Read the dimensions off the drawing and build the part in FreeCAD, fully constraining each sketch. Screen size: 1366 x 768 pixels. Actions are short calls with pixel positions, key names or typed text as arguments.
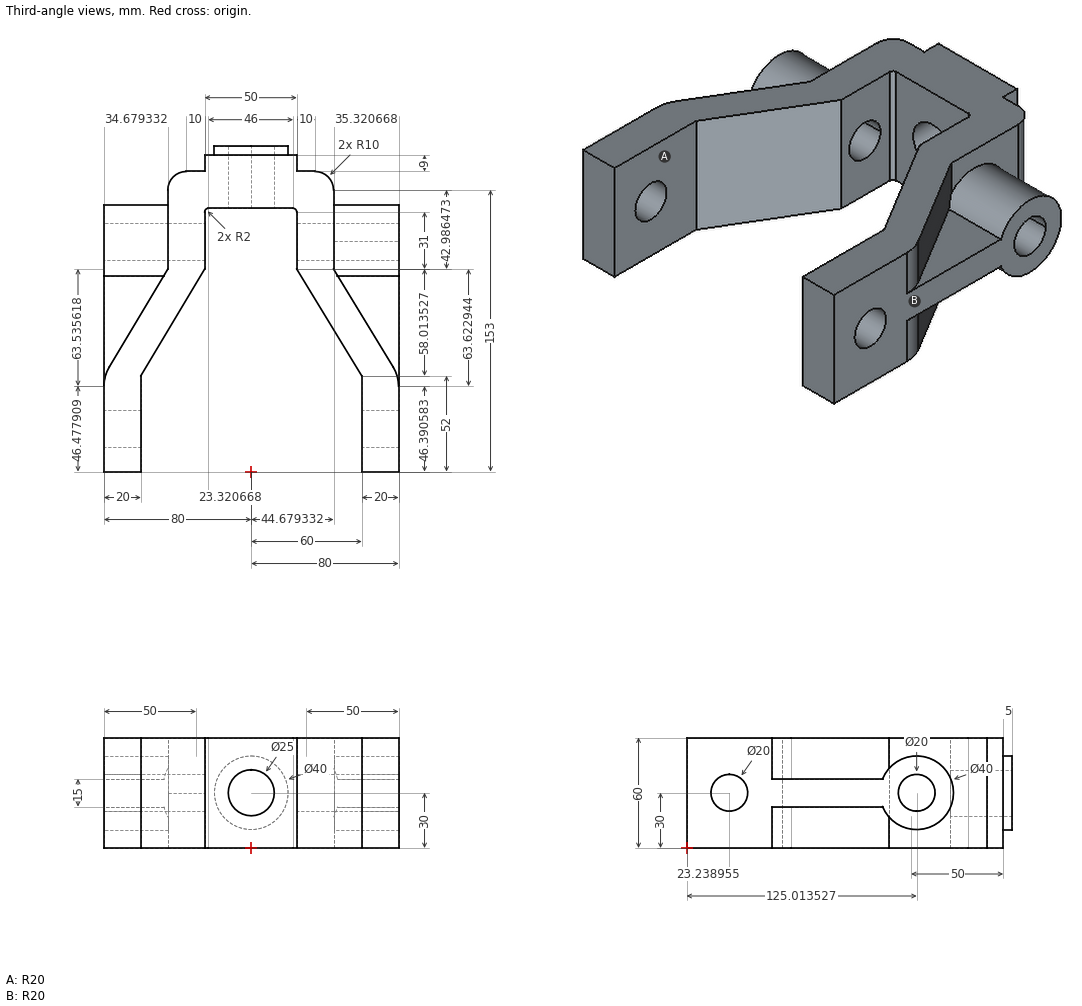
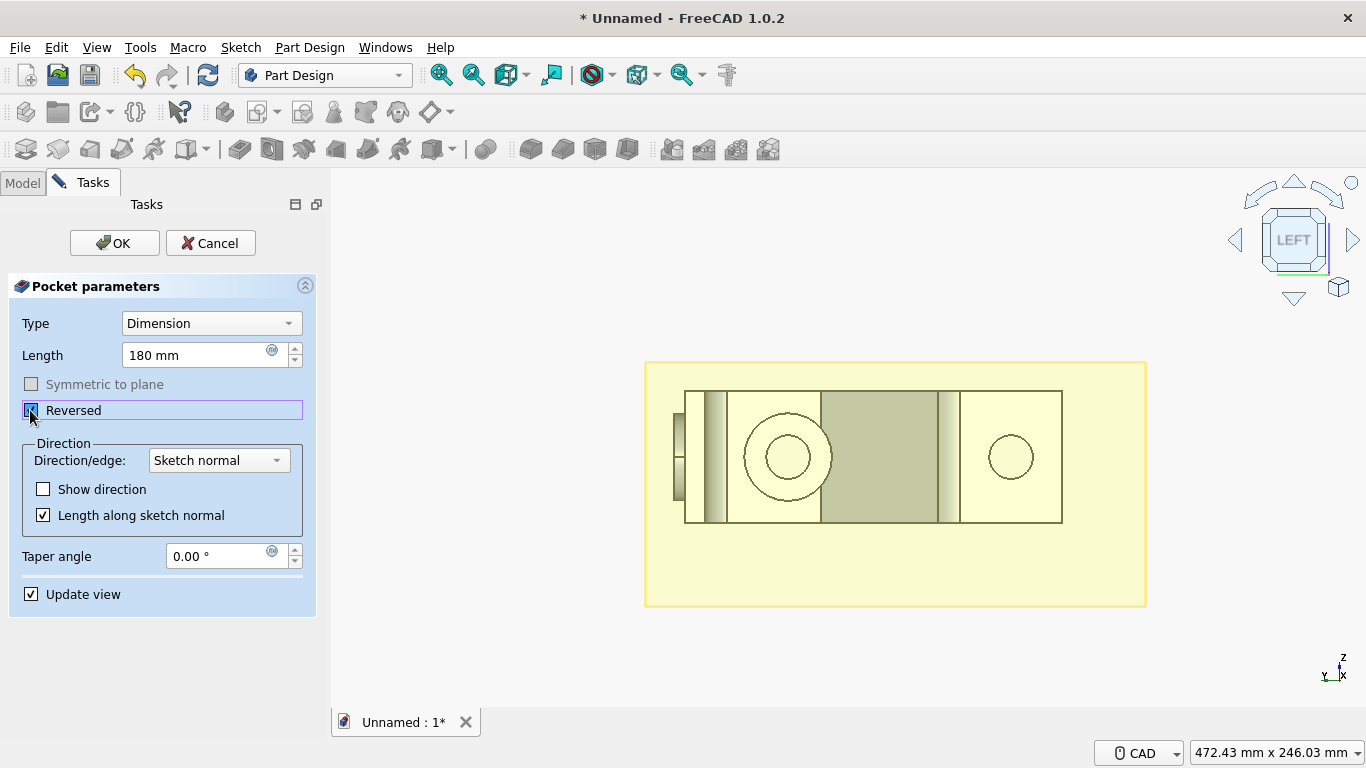
click(115, 243)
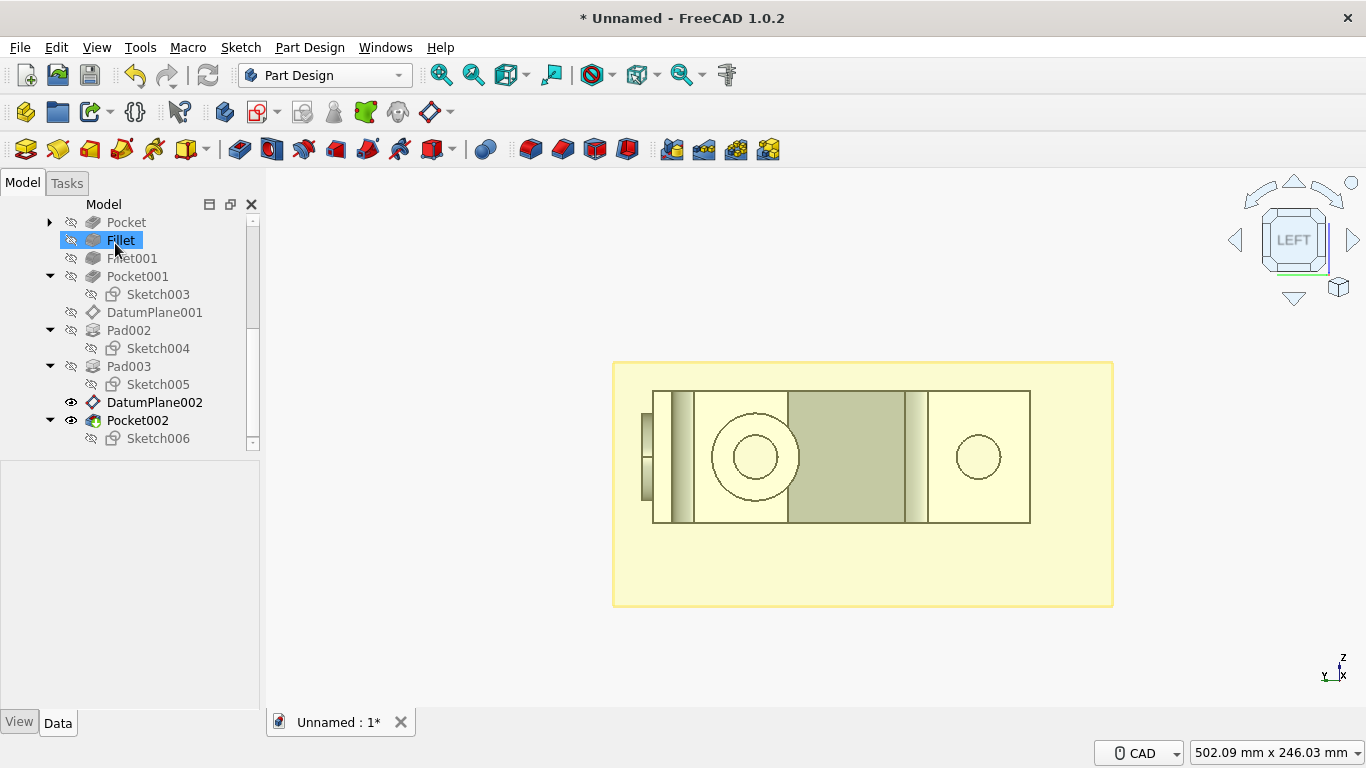
click(116, 402)
key(space)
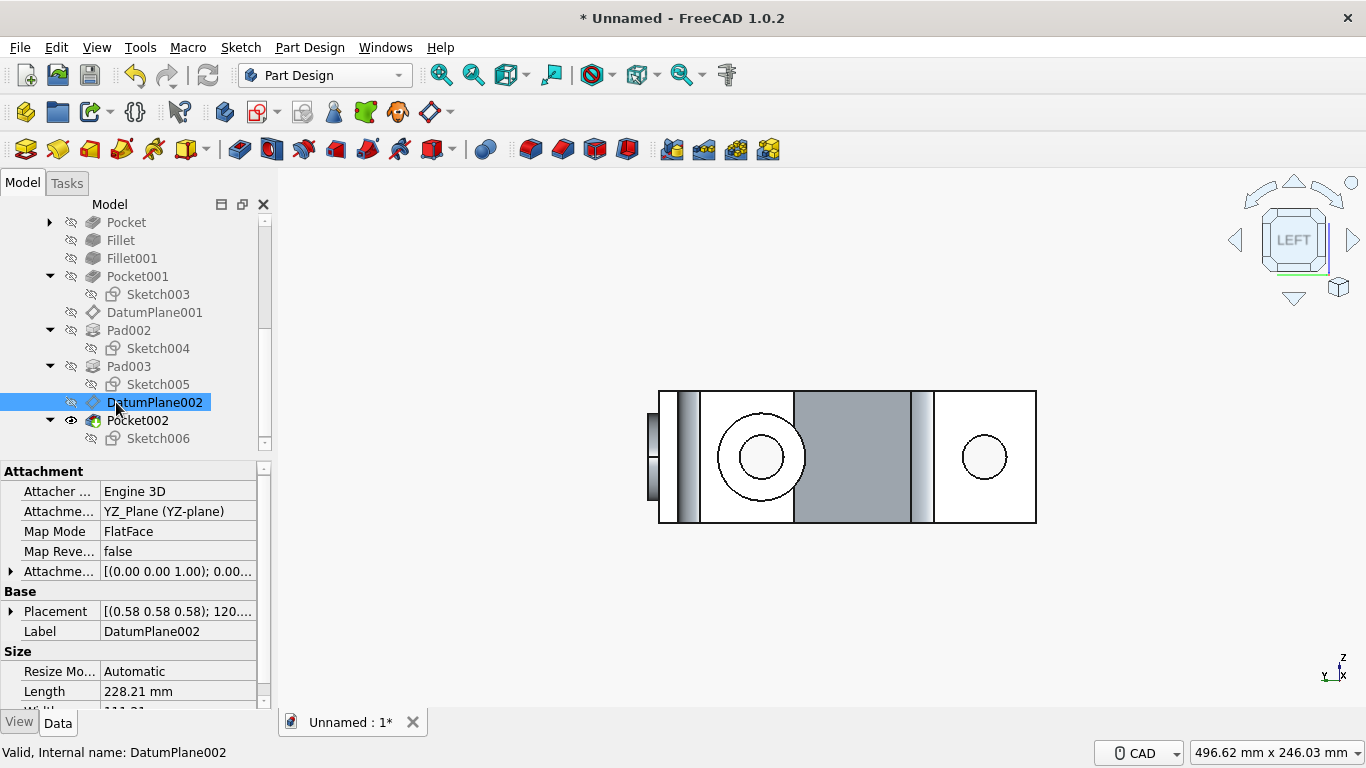
key(v)
key(f)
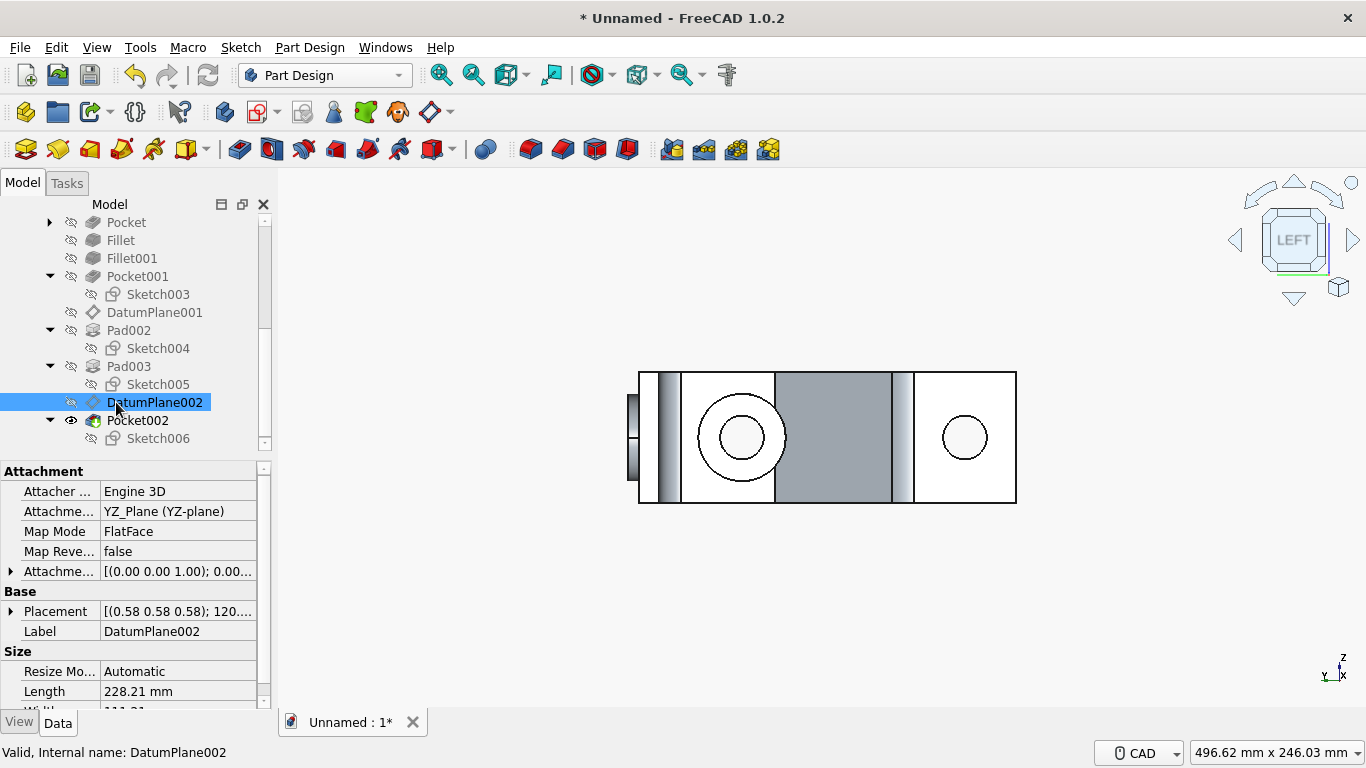
scroll(140, 326, down, 3)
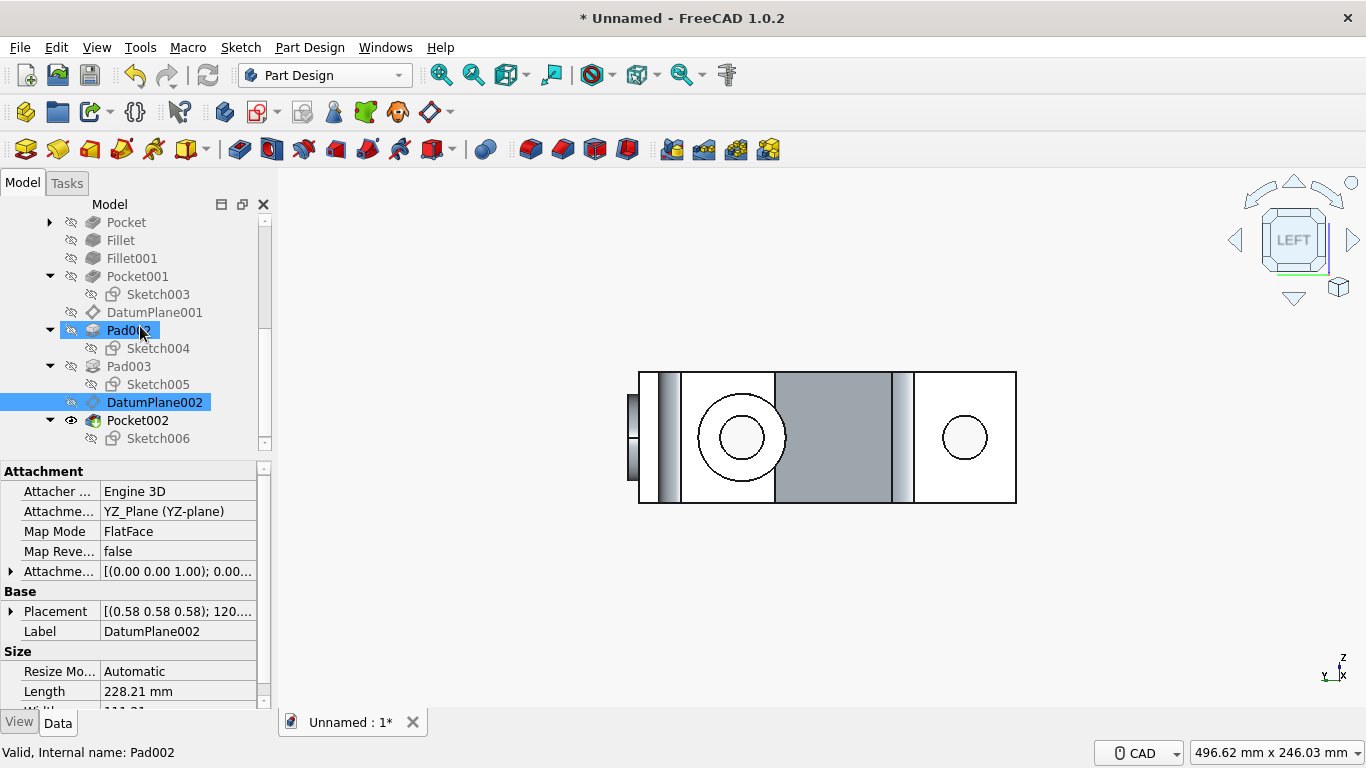
scroll(140, 326, up, 15)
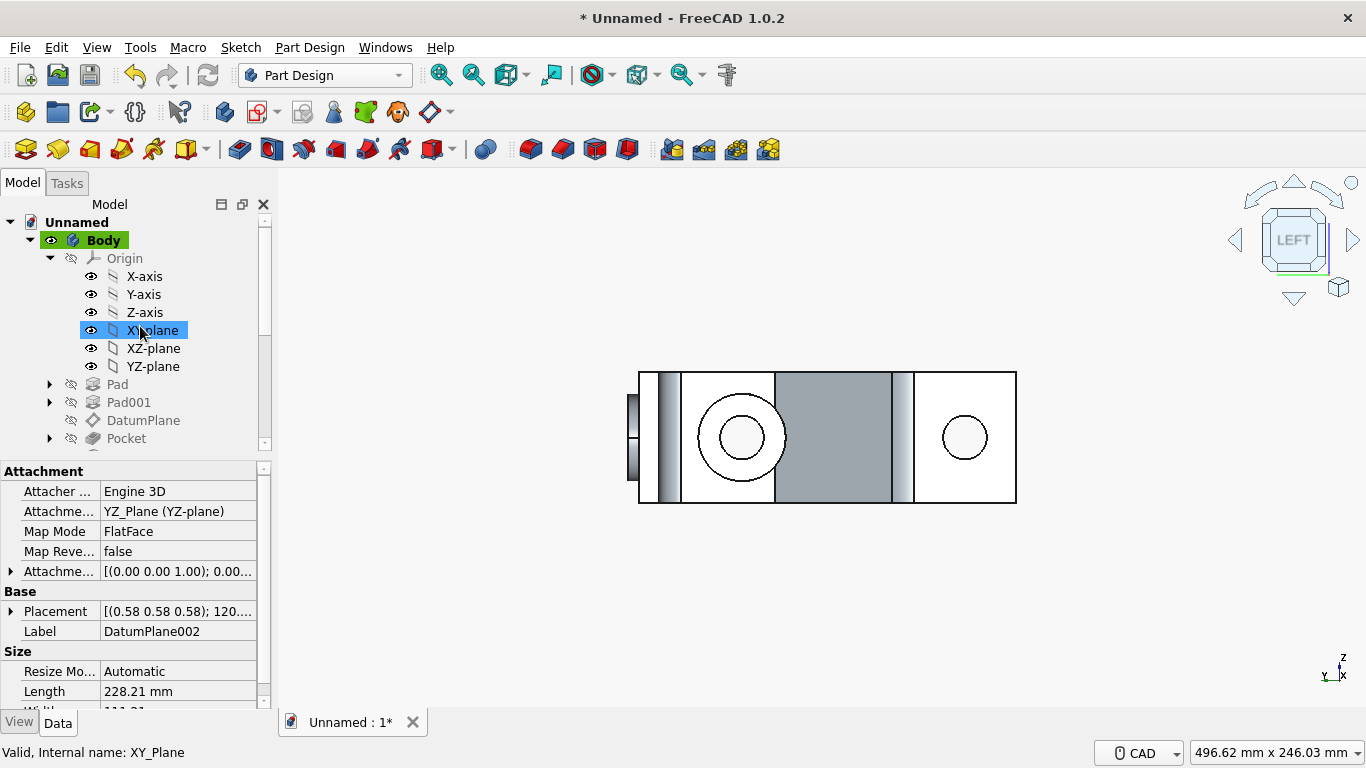
click(136, 330)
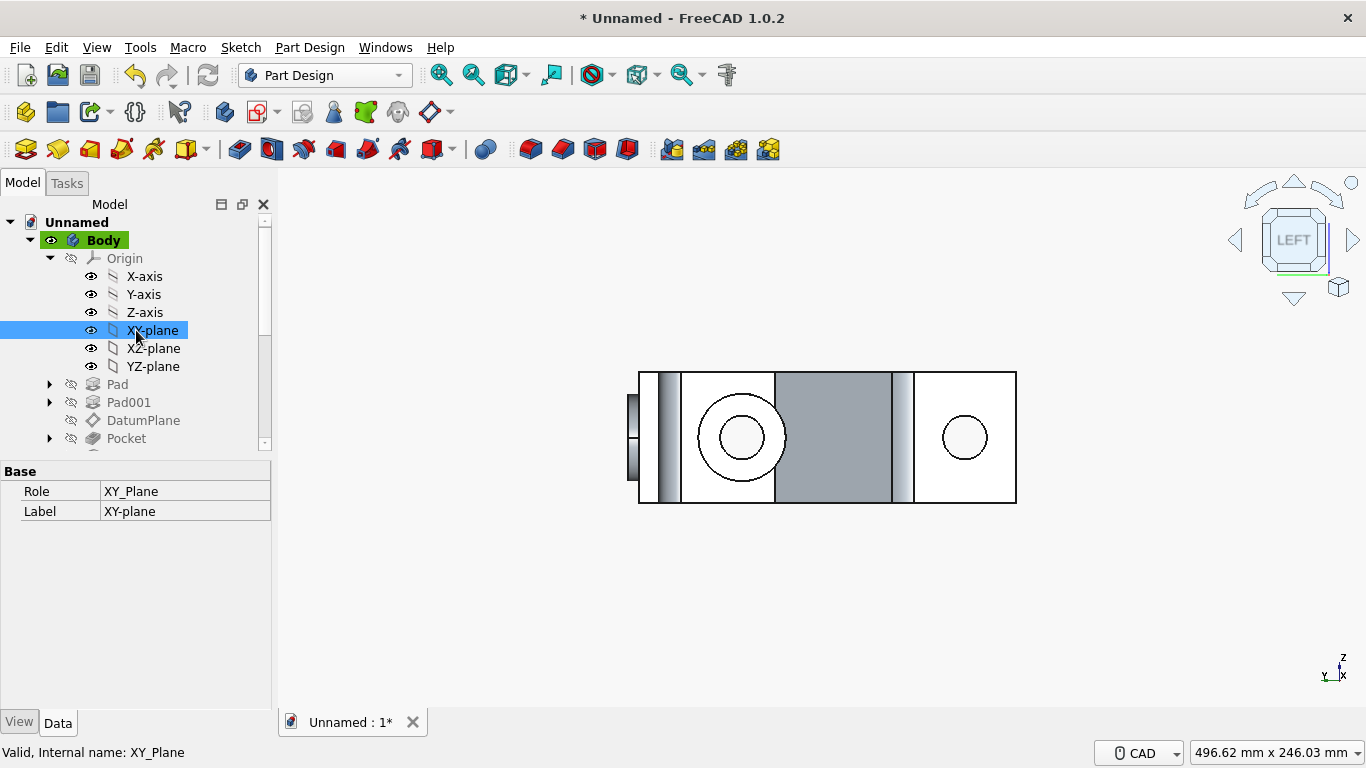
click(430, 112)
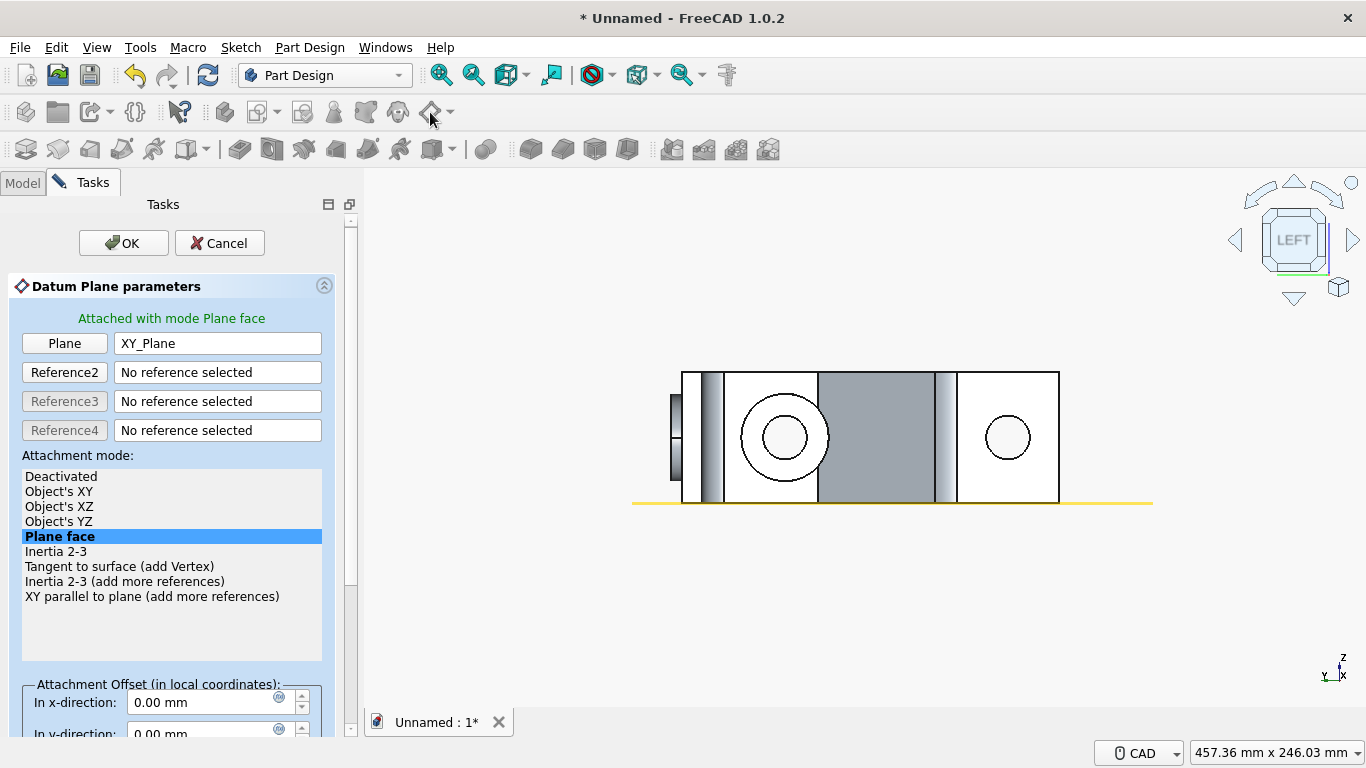
scroll(351, 475, down, 2)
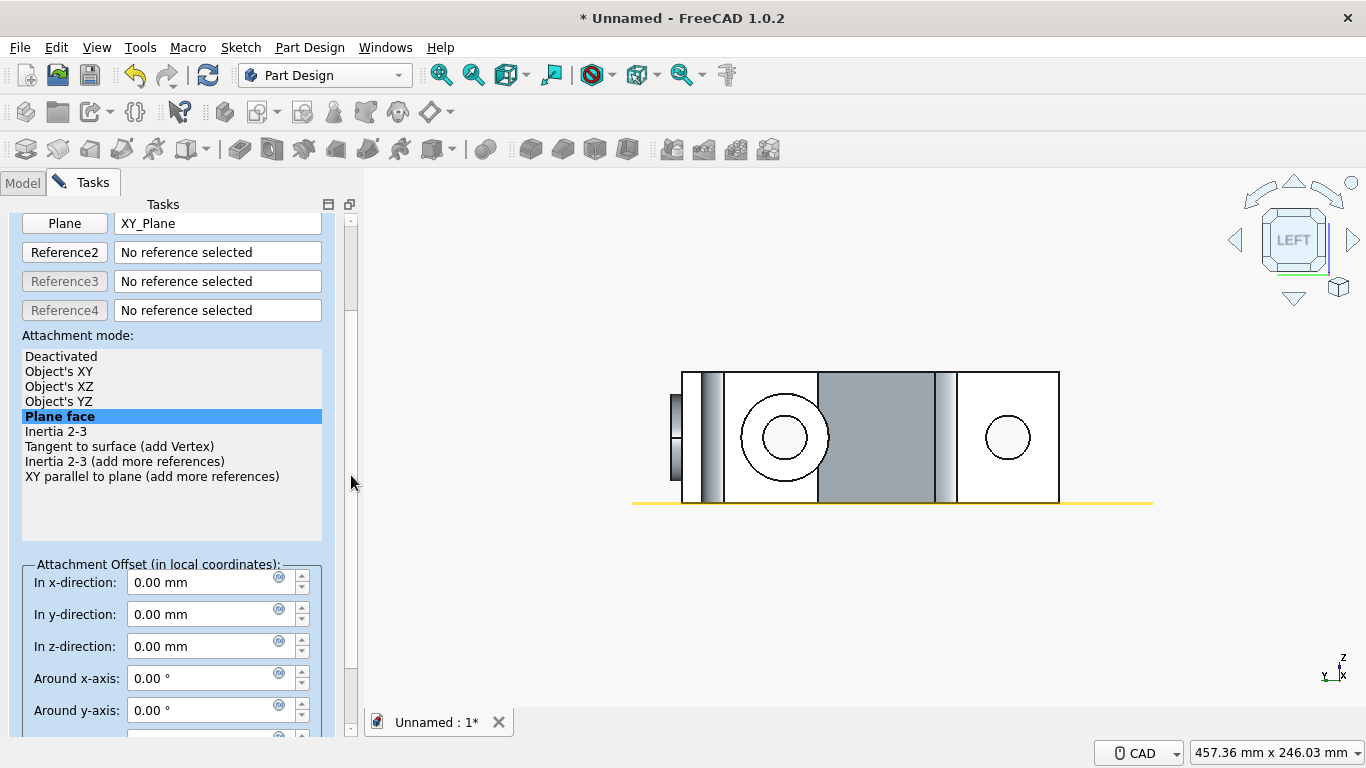
triple_click(210, 646)